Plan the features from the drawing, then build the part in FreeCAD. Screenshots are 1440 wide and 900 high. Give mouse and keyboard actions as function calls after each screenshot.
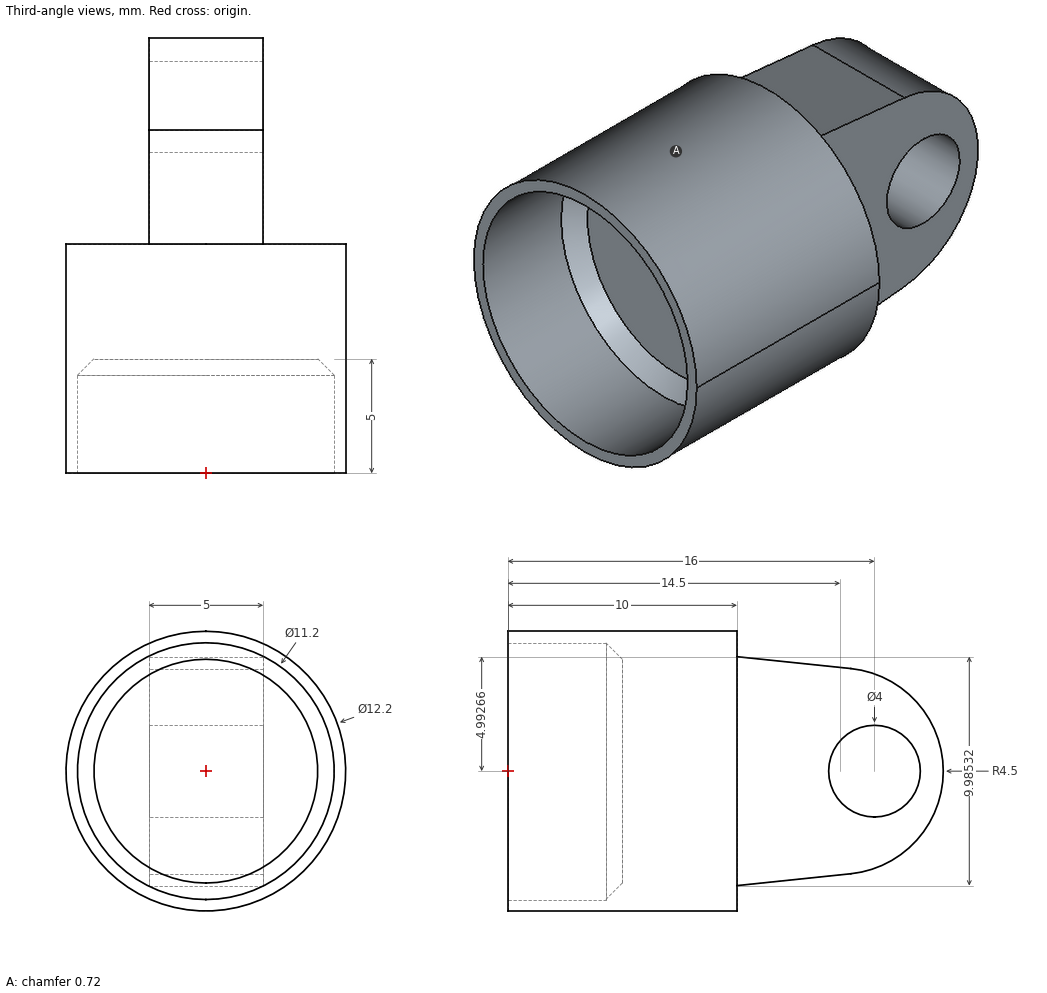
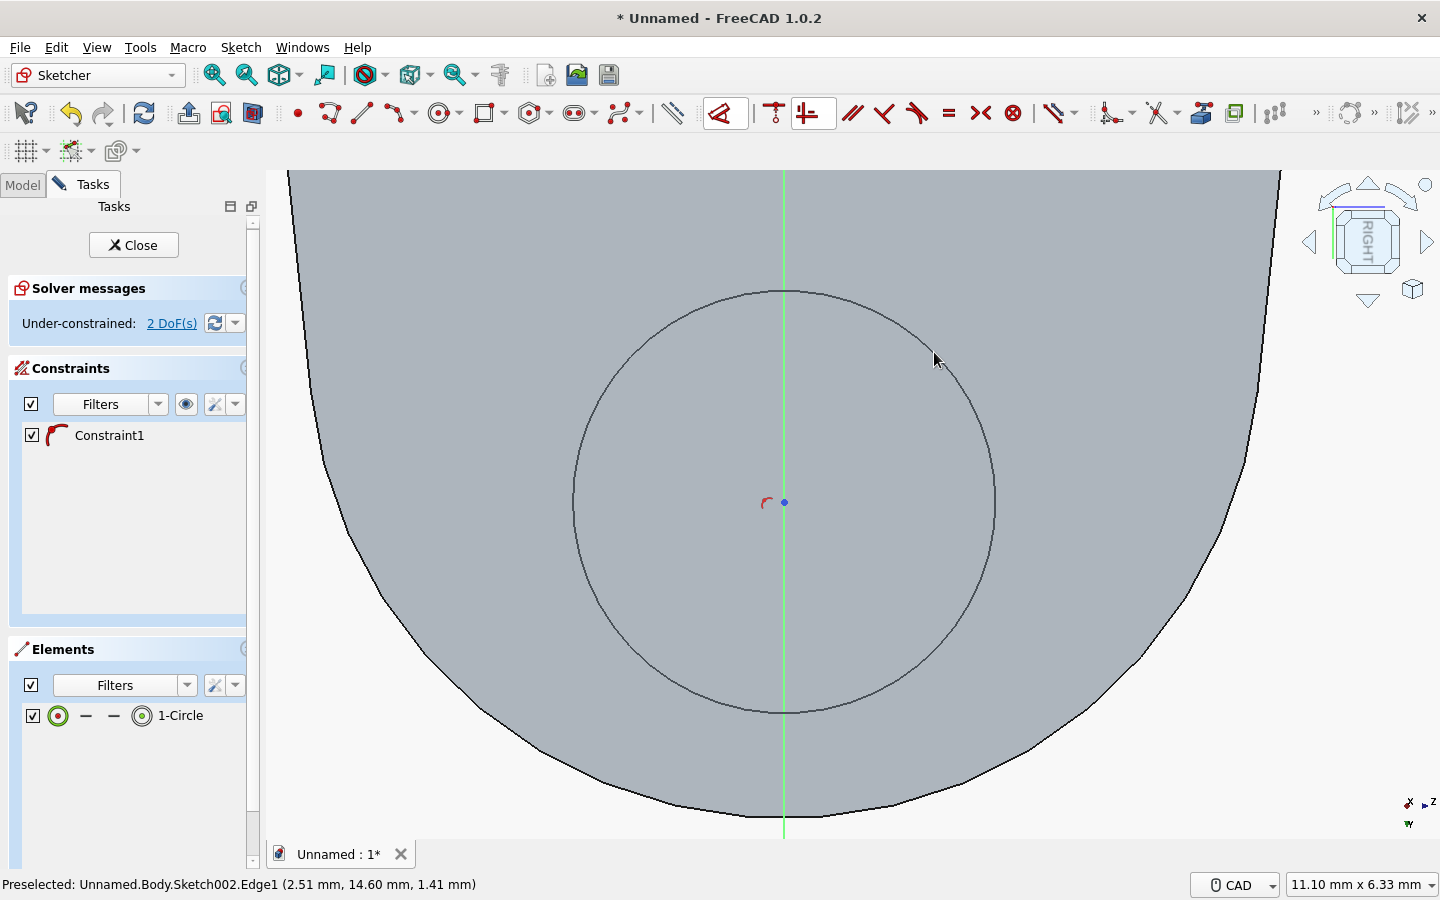
key(d)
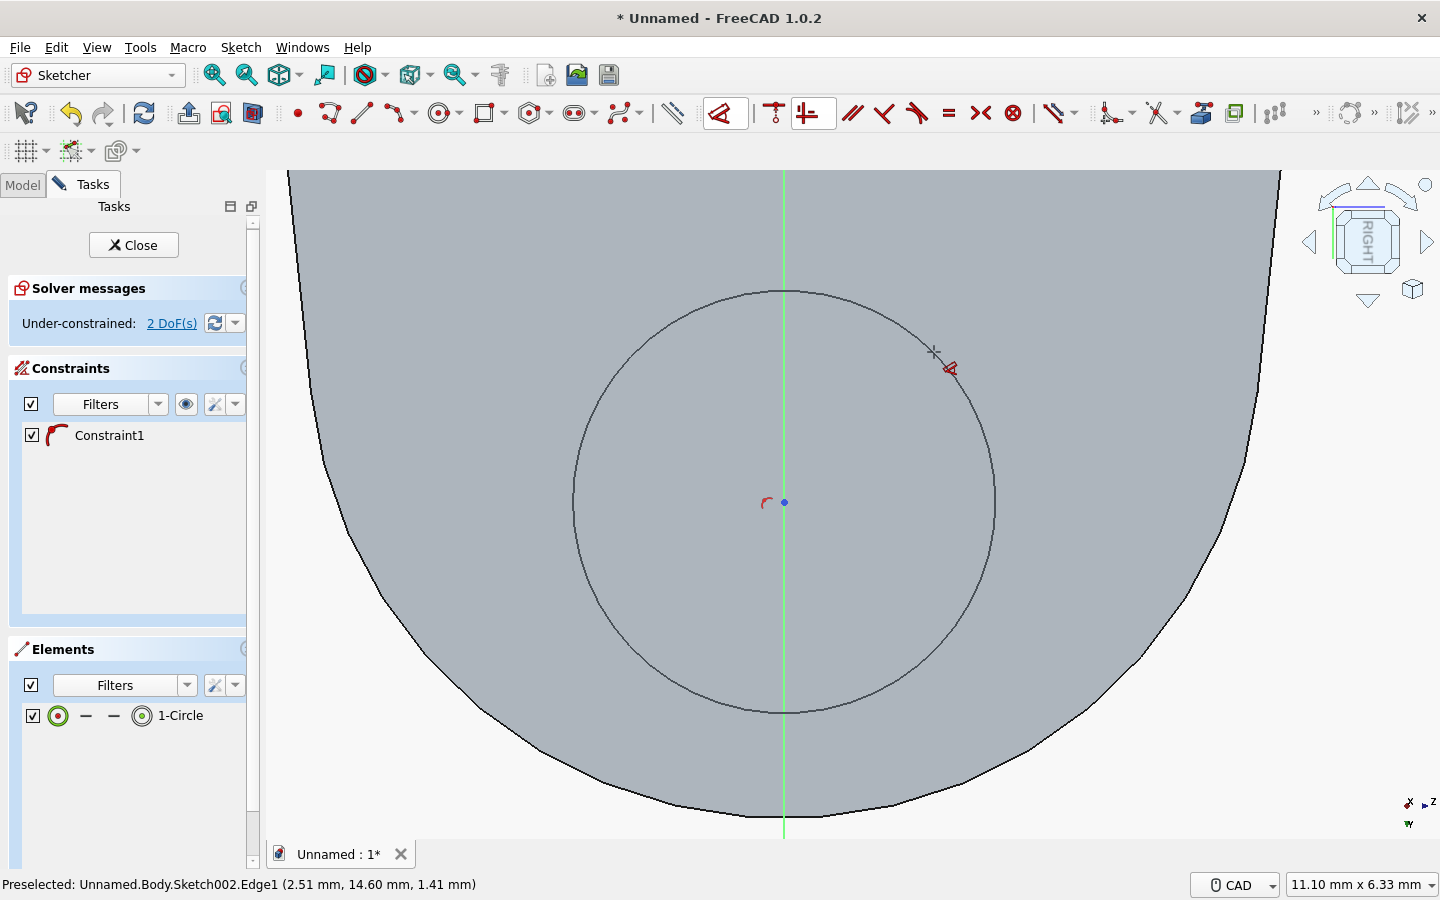
click(933, 352)
click(956, 329)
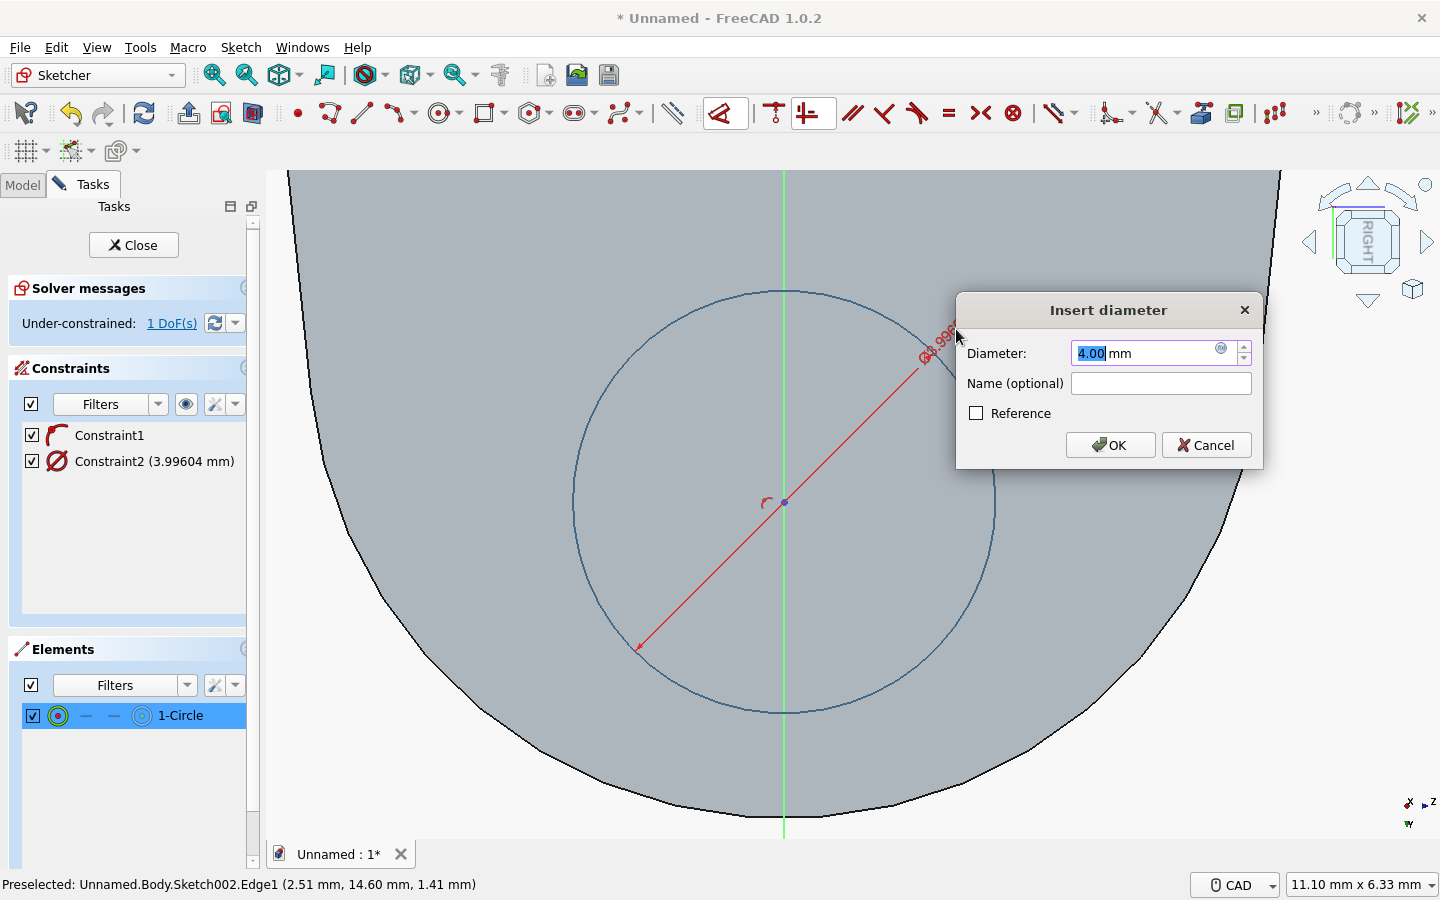
text(4)
key(Return)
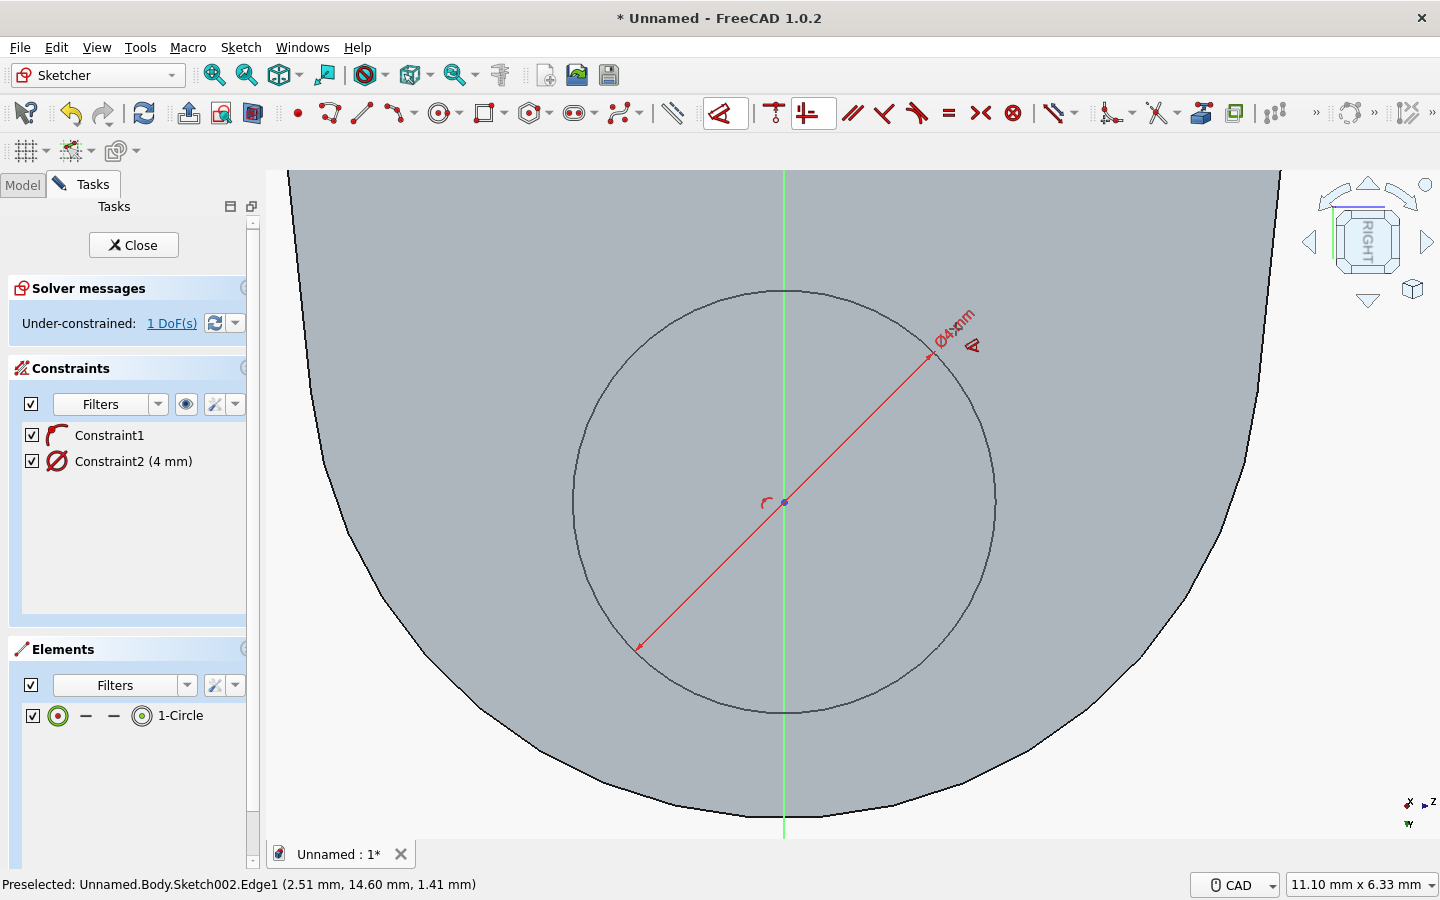
click(784, 502)
click(818, 350)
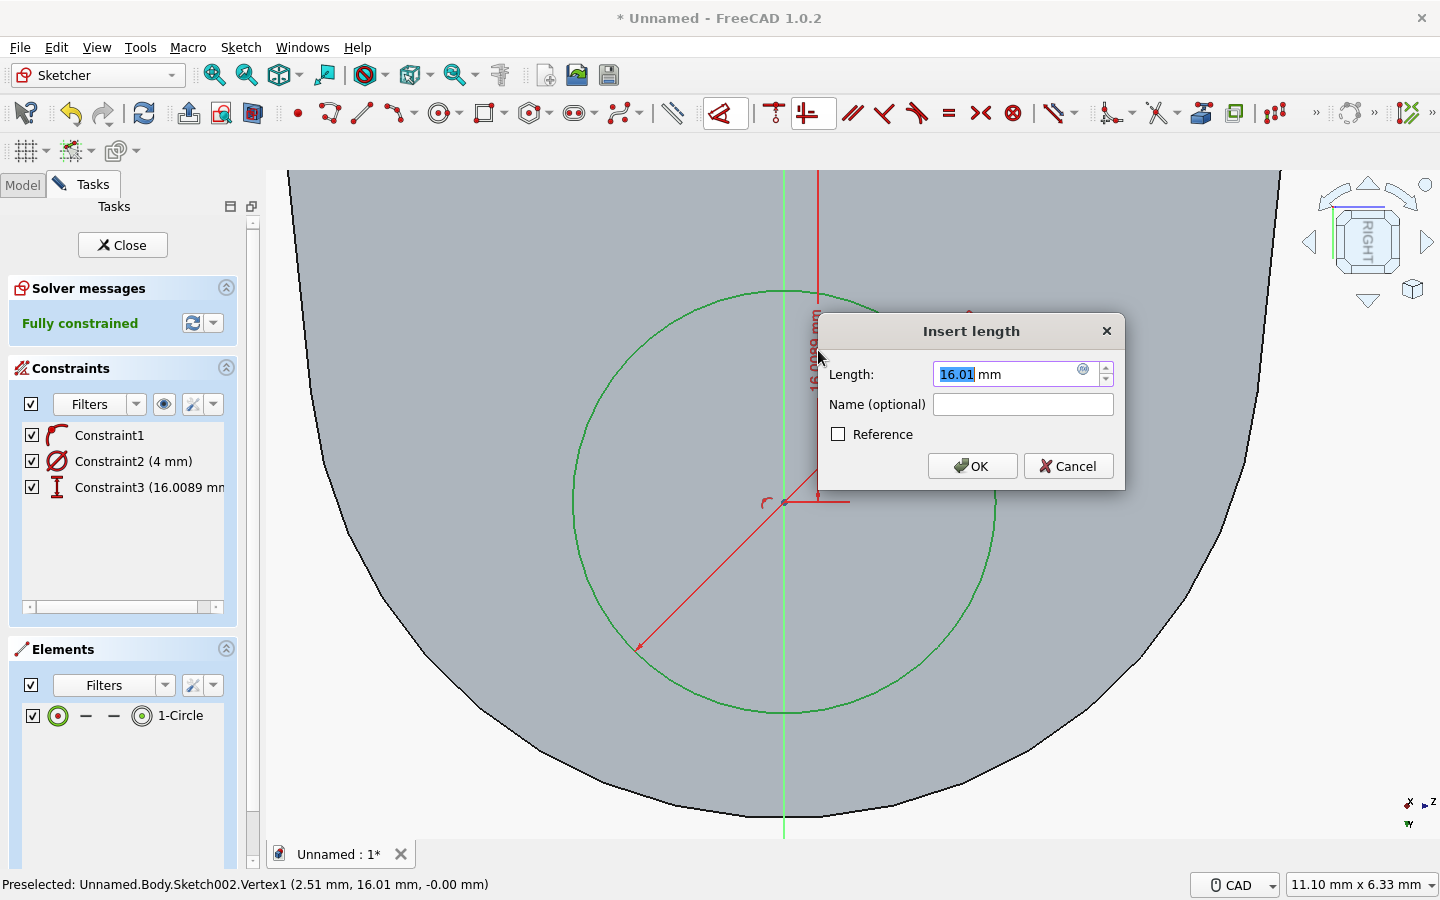
text(16)
key(Return)
key(Escape)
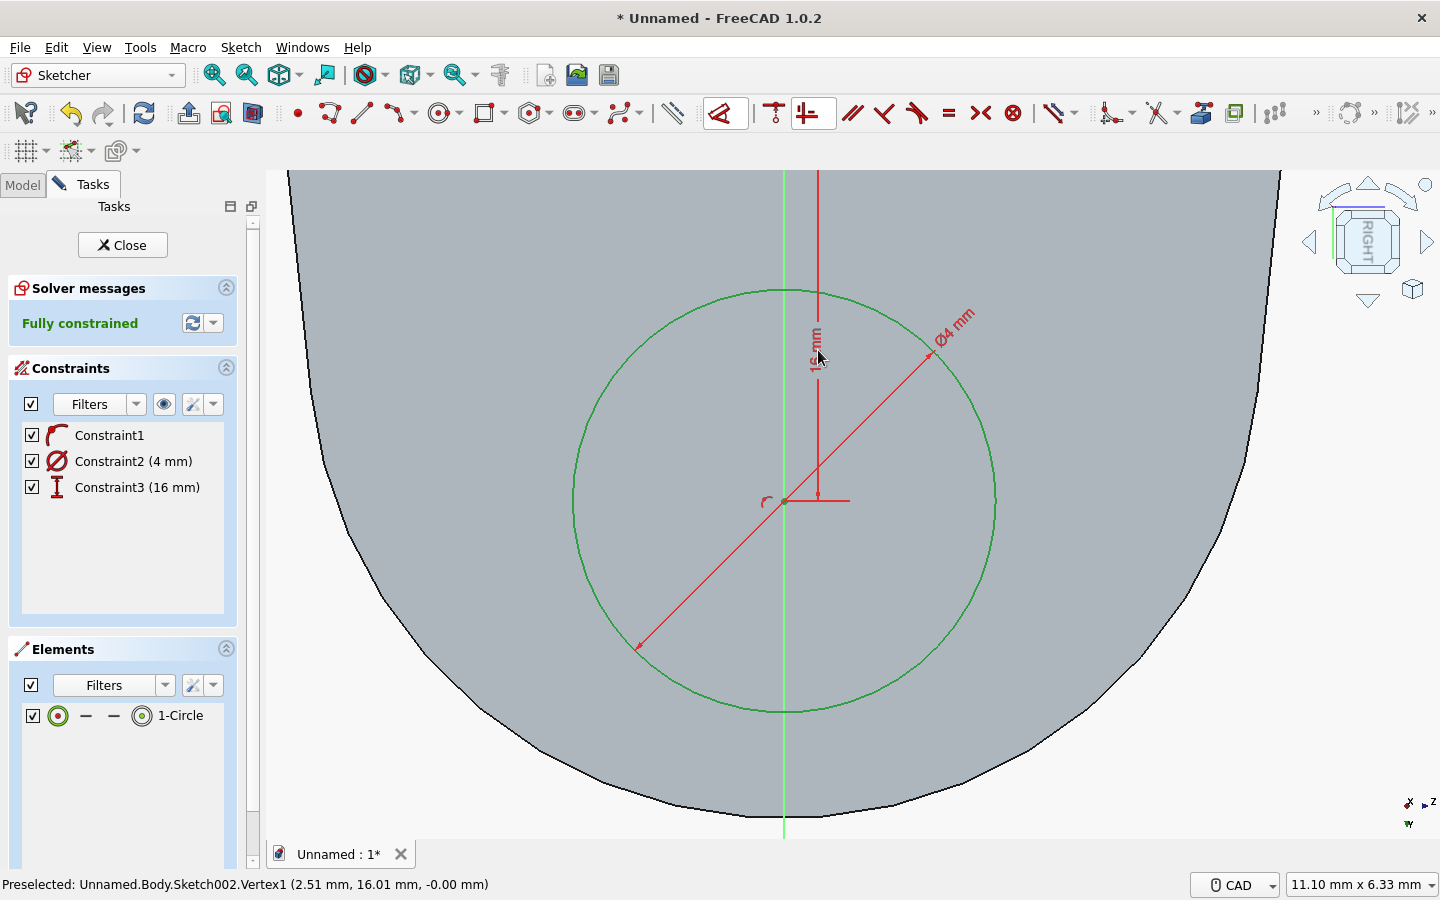
click(123, 245)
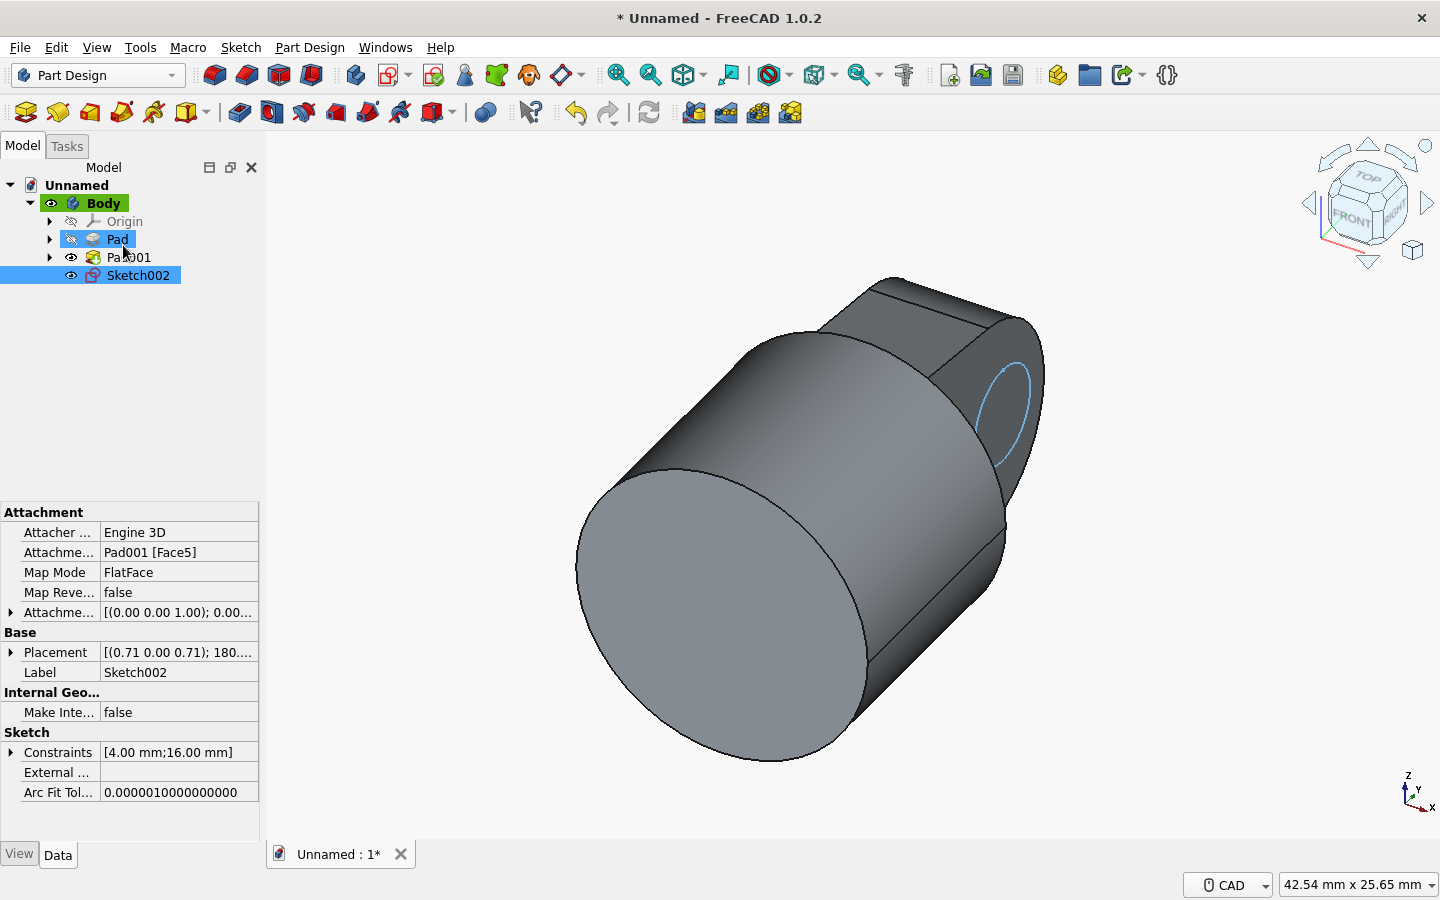
click(240, 112)